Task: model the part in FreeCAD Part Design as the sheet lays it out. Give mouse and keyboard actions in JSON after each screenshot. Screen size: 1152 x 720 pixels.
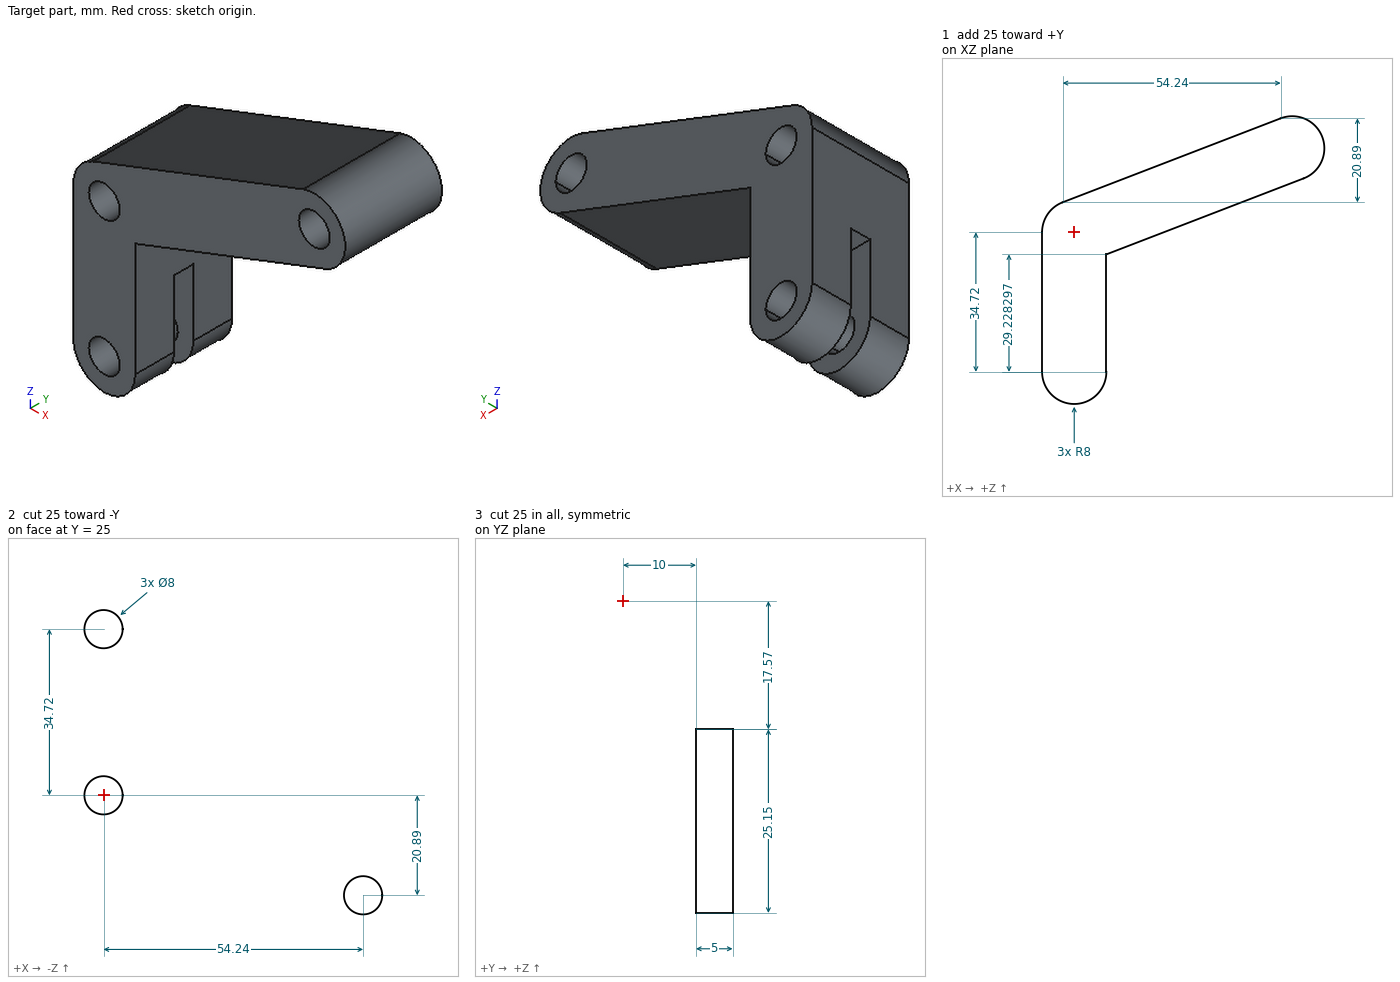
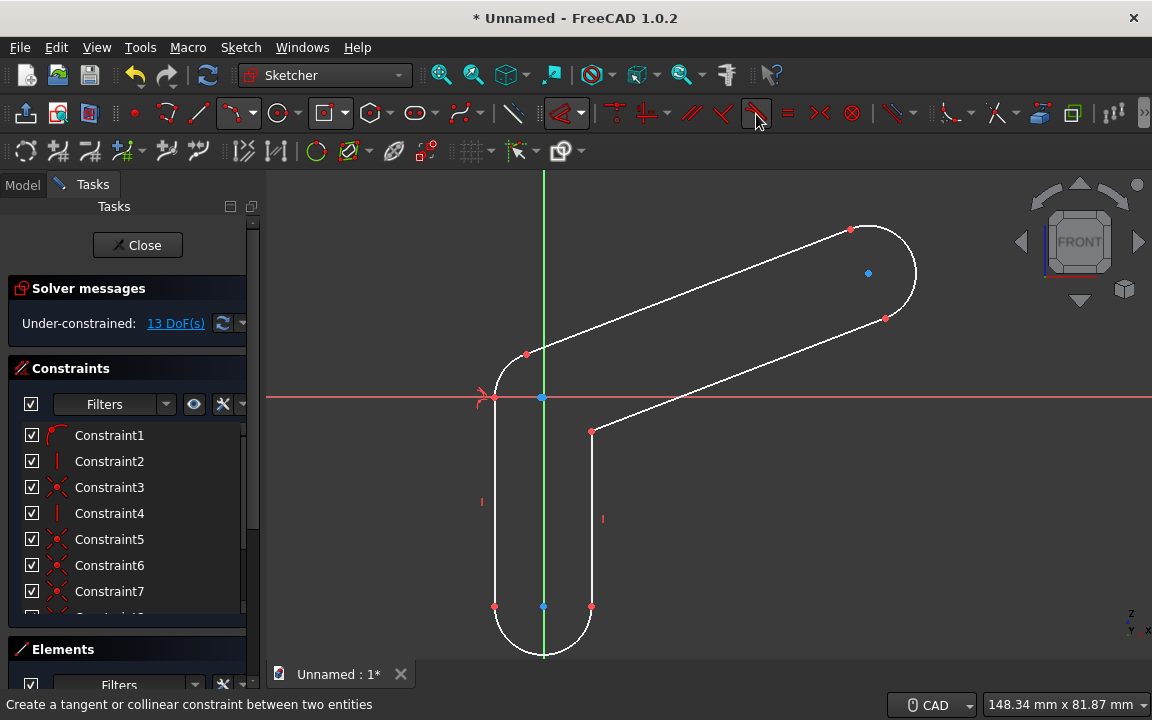
{"action": "left_click", "coordinate": [495, 544]}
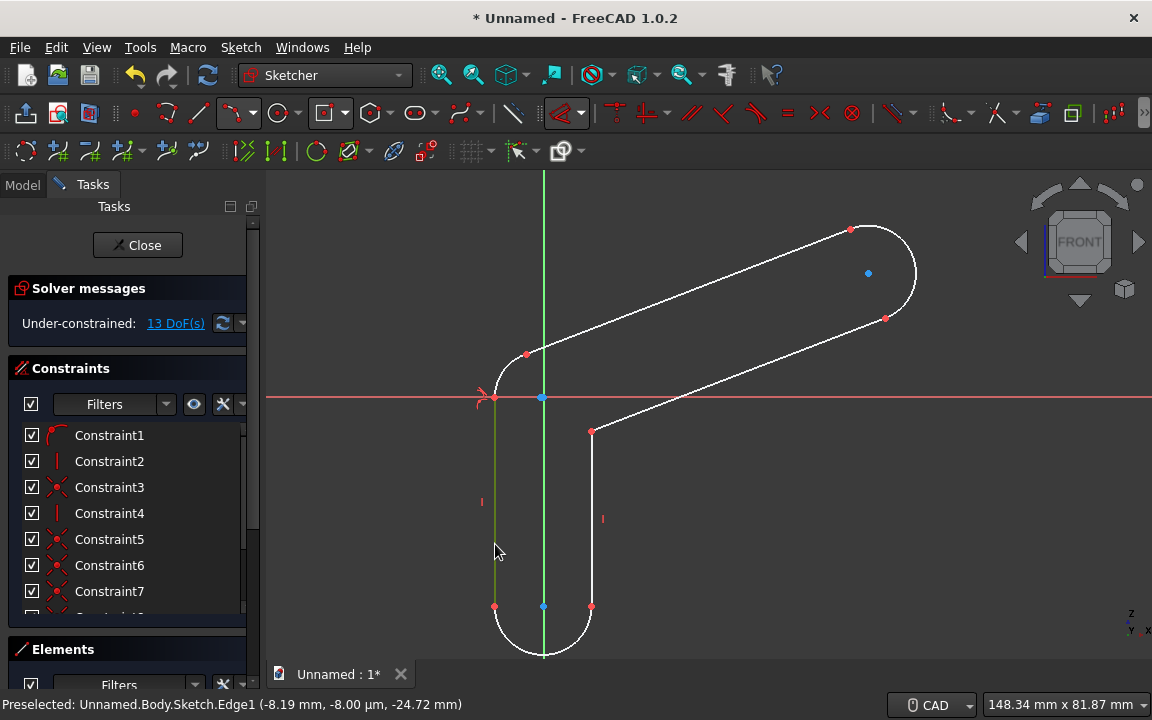
{"action": "scroll", "coordinate": [511, 362], "scroll_direction": "down", "scroll_amount": 2}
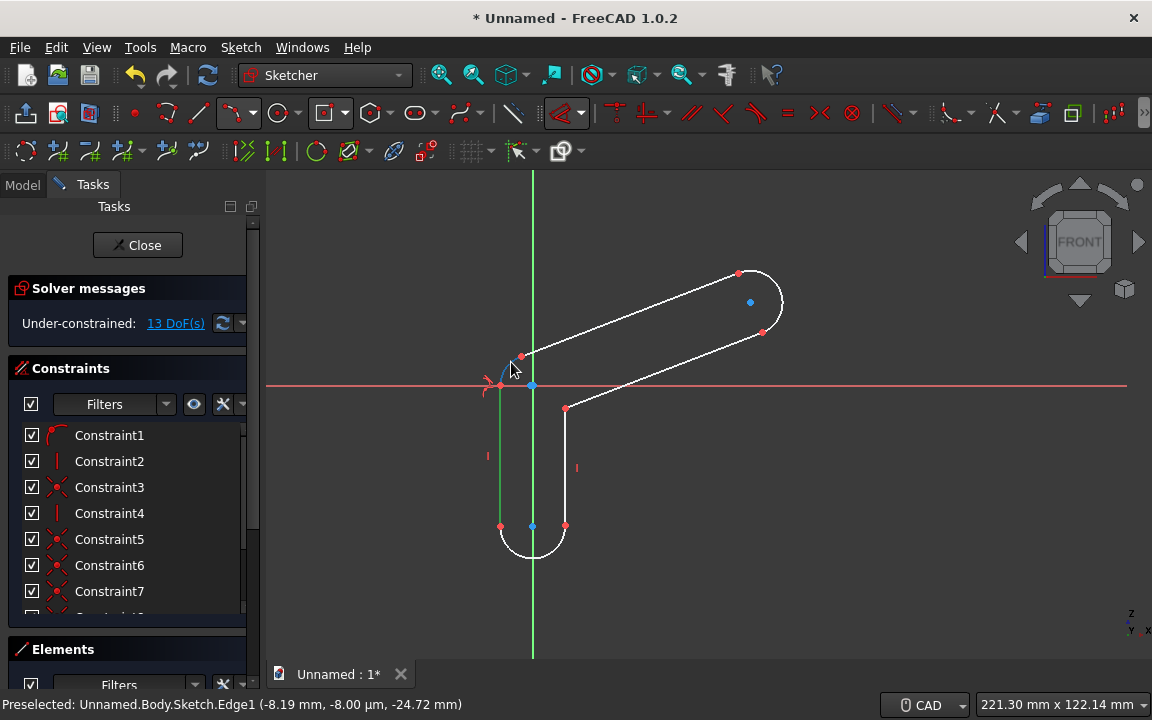
{"action": "left_click", "coordinate": [514, 552]}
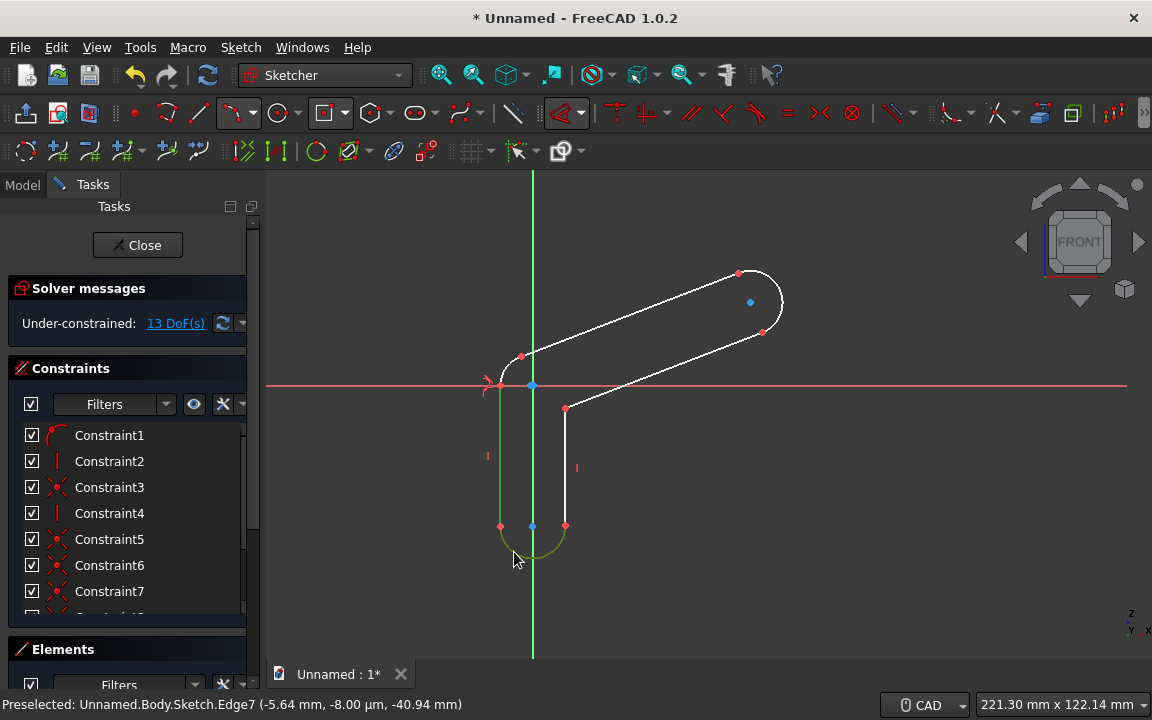
{"action": "left_click", "coordinate": [756, 114]}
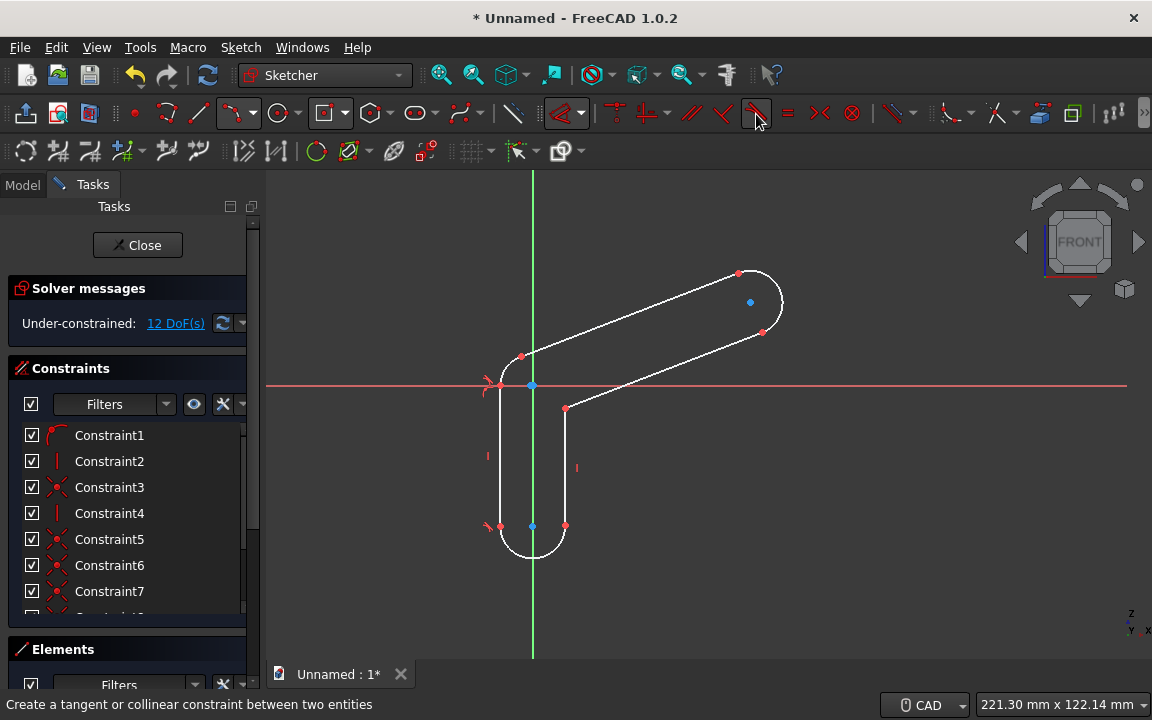
{"action": "left_click", "coordinate": [587, 332]}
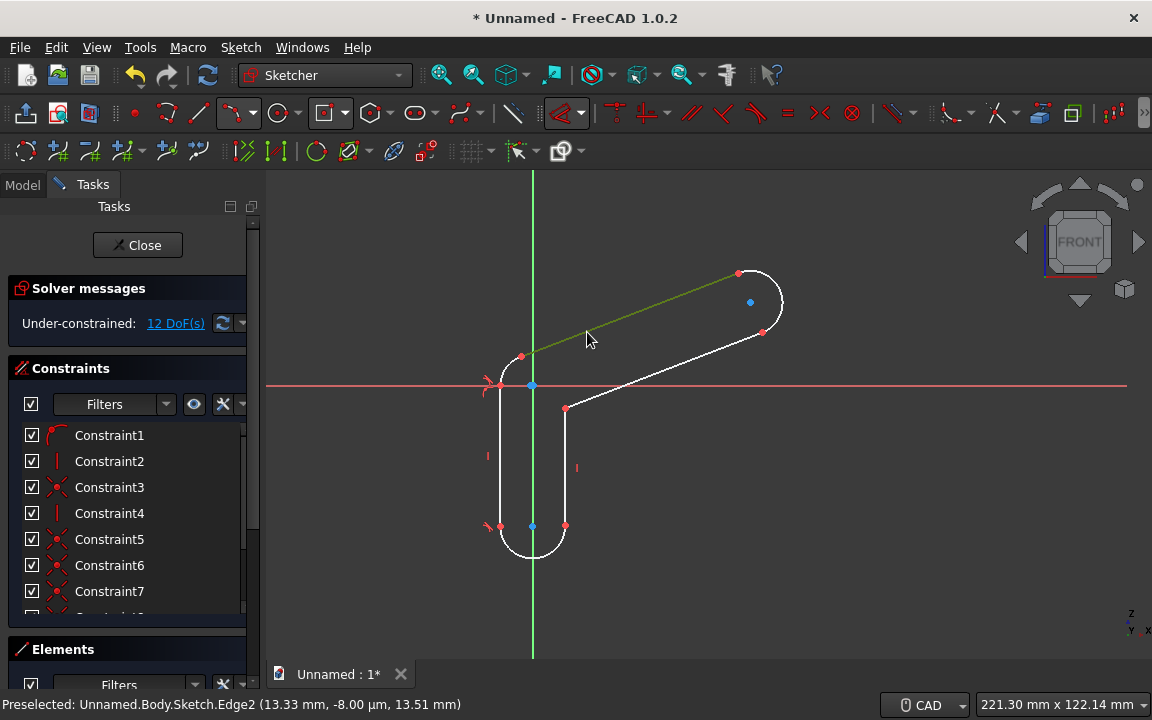
{"action": "left_click", "coordinate": [511, 362]}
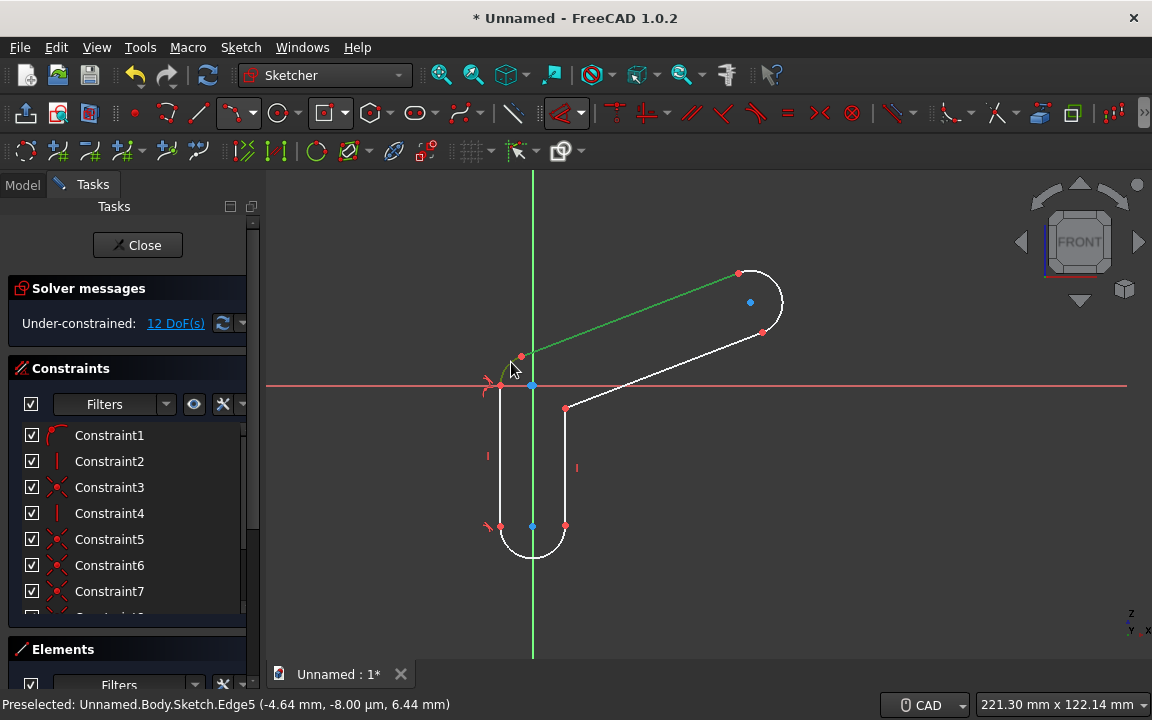
{"action": "key", "text": "t"}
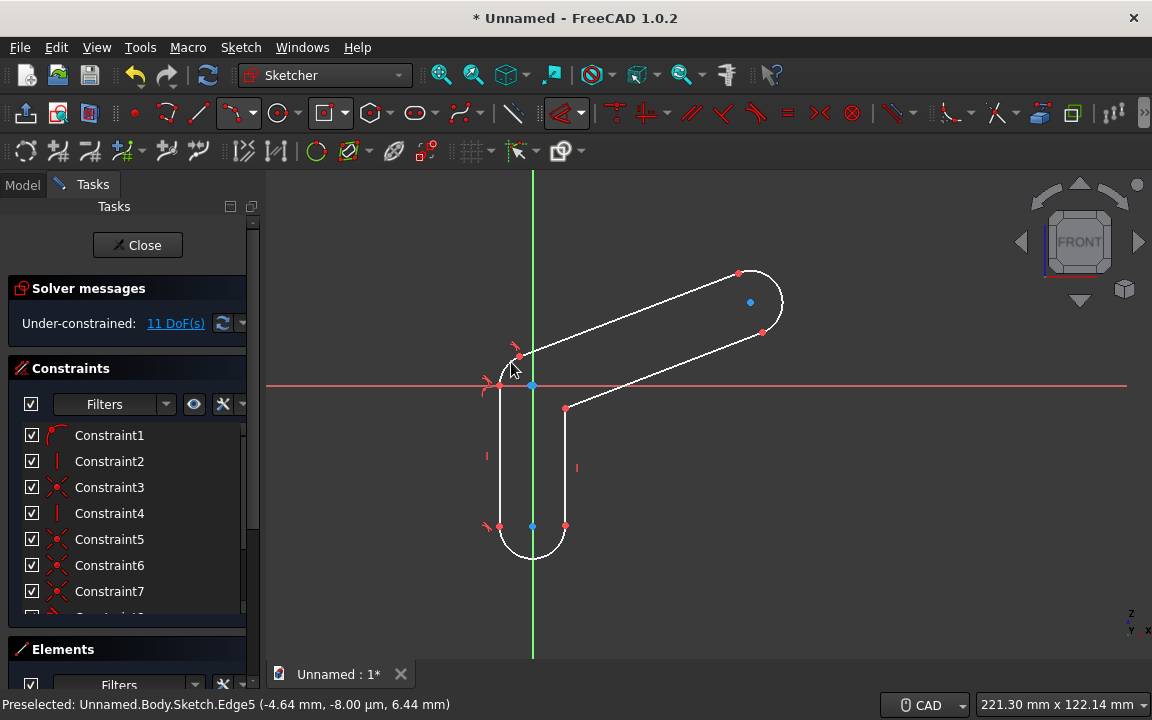
{"action": "left_click", "coordinate": [585, 332]}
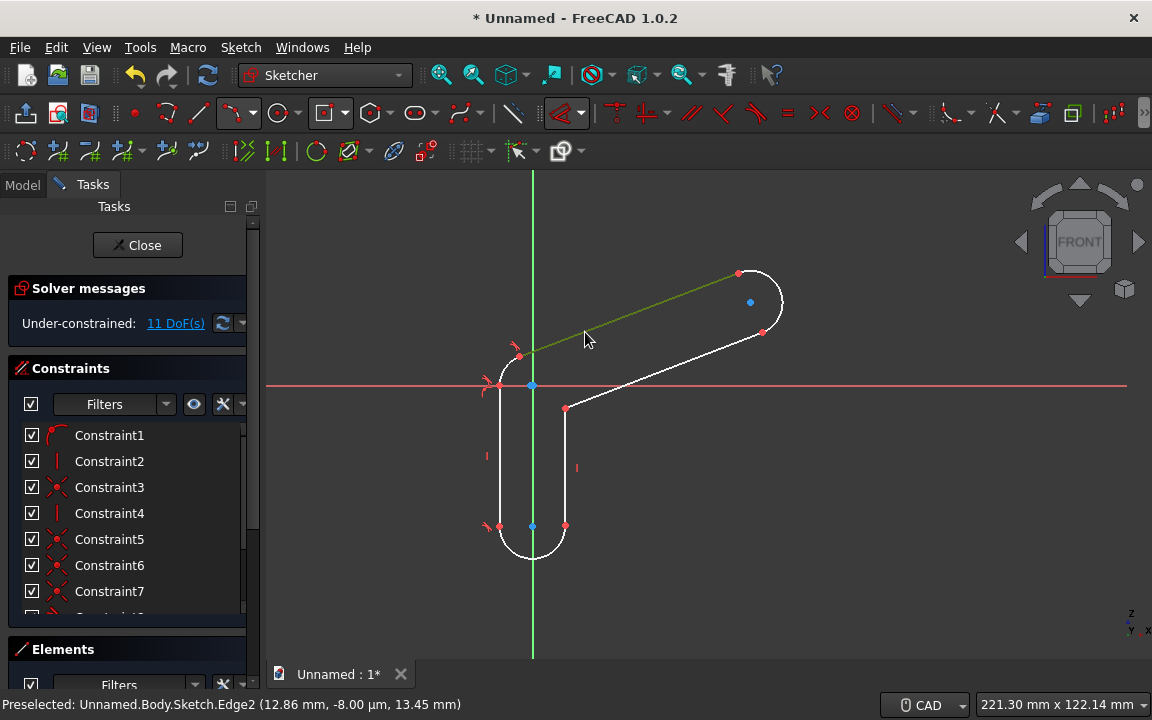
{"action": "left_click", "coordinate": [782, 311]}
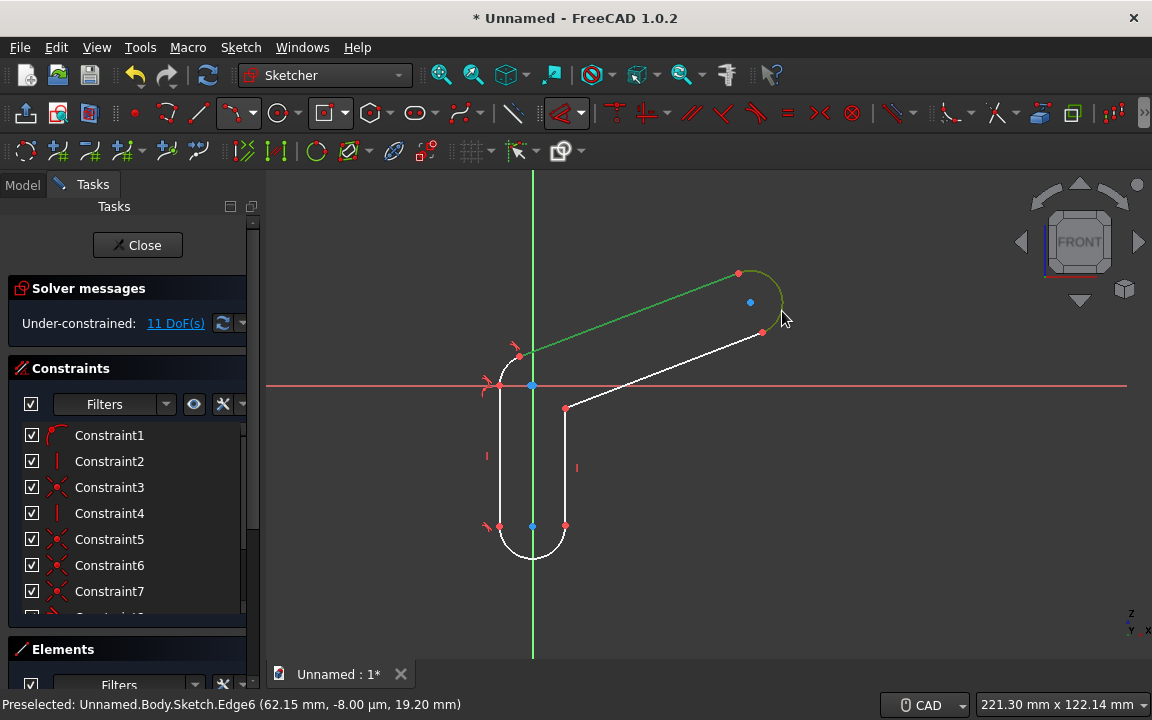
{"action": "left_click", "coordinate": [756, 114]}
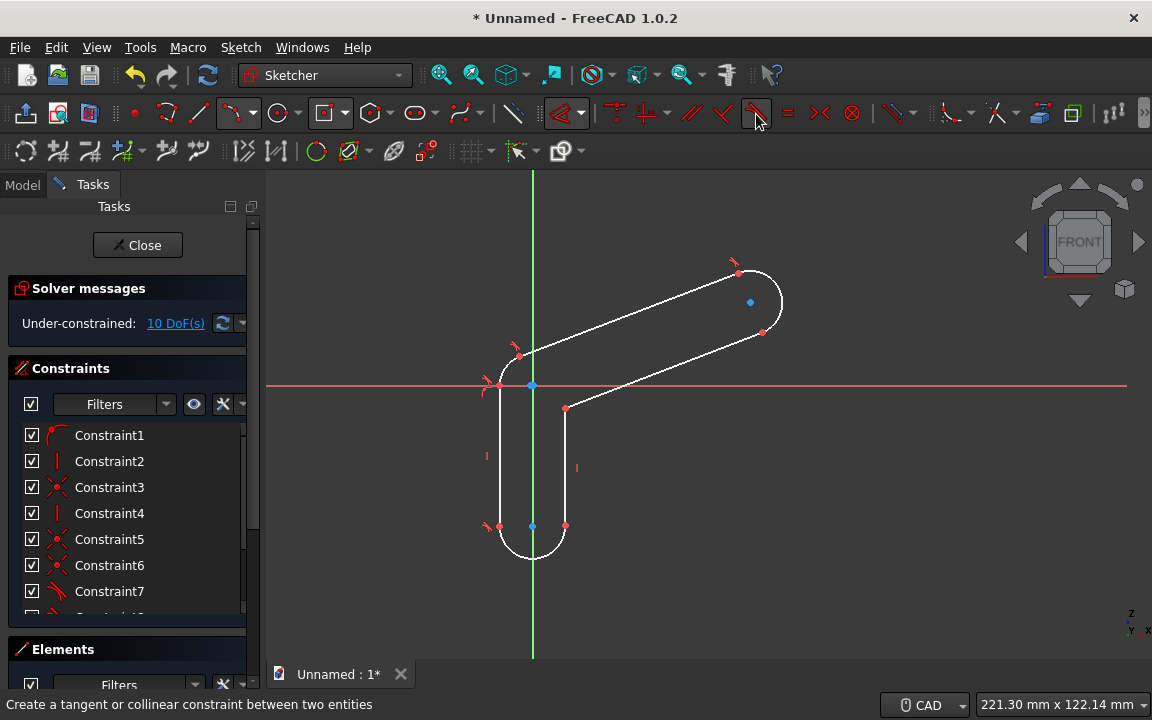
{"action": "left_click", "coordinate": [703, 355]}